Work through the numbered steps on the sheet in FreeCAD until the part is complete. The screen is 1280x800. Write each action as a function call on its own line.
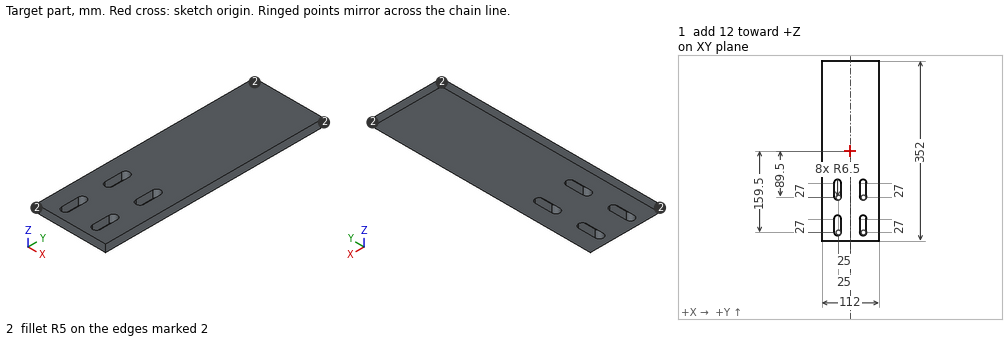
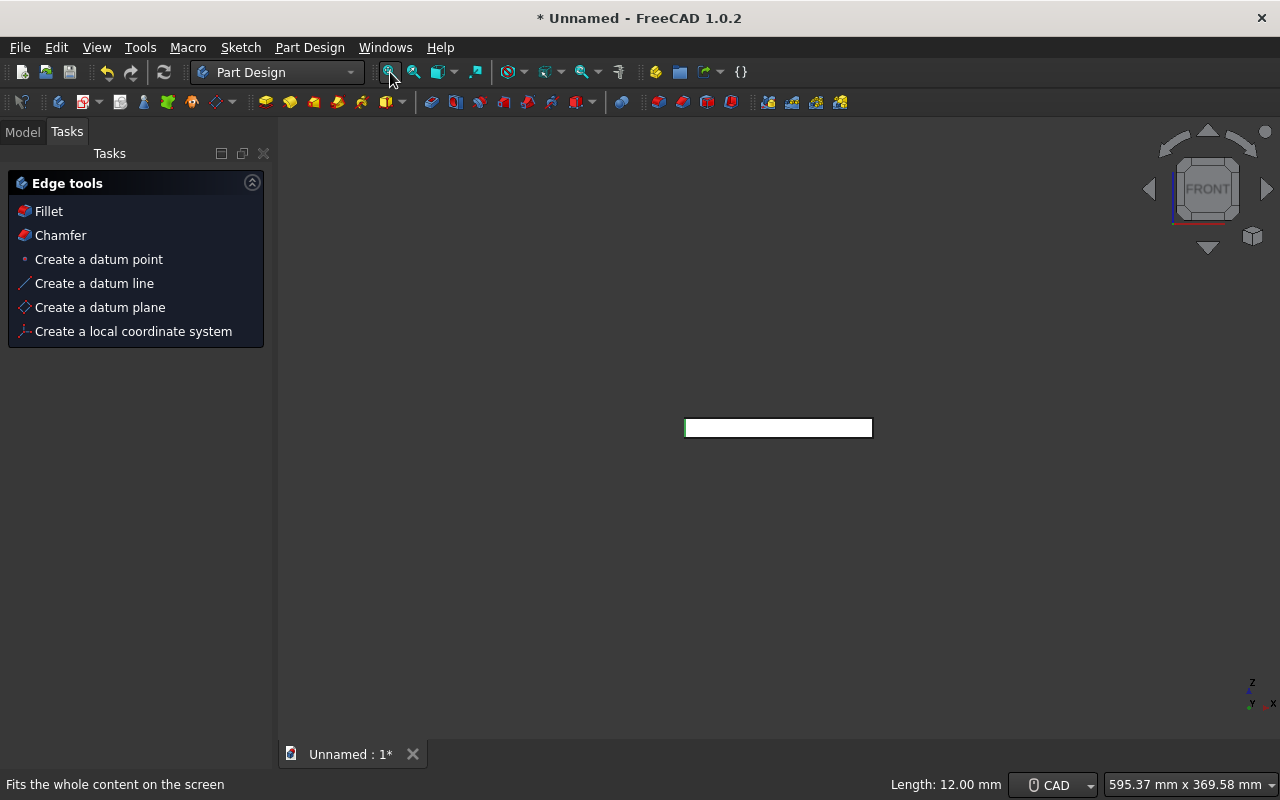
key(3)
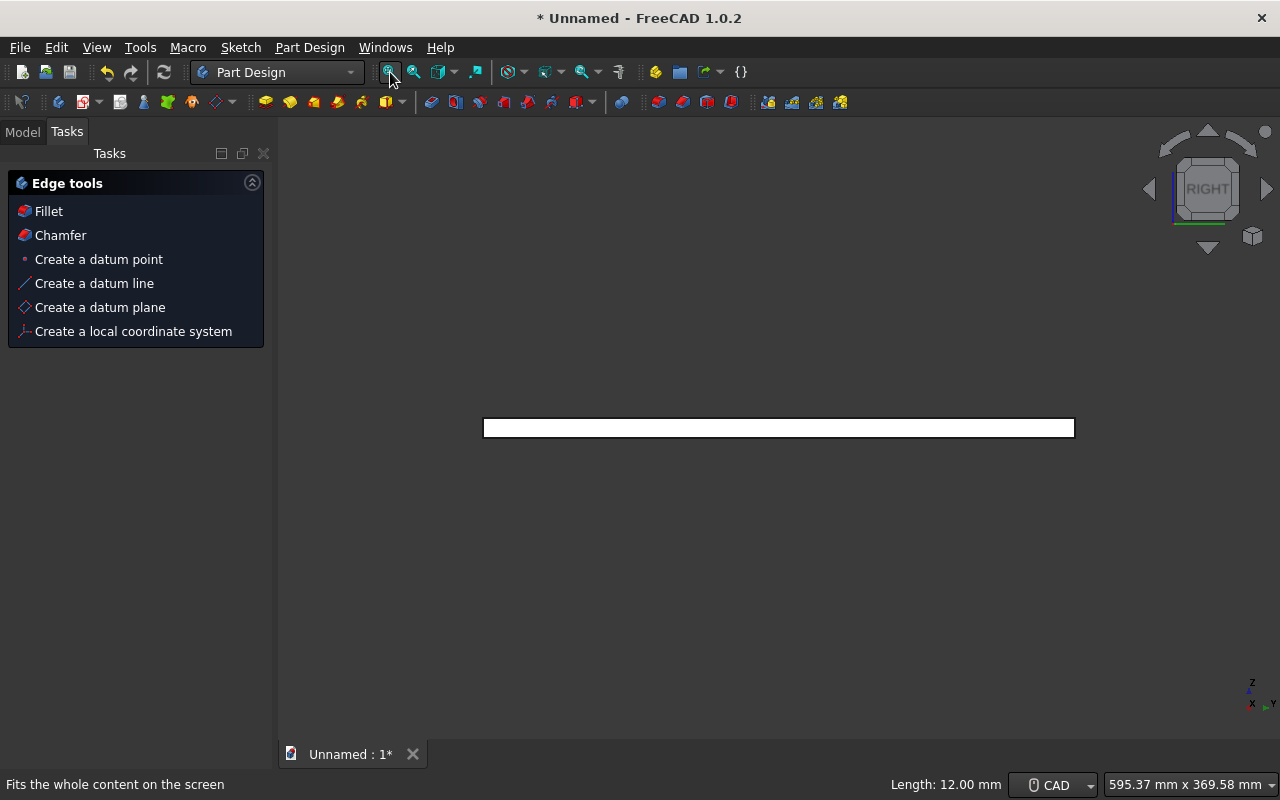
click(1075, 427, ctrl)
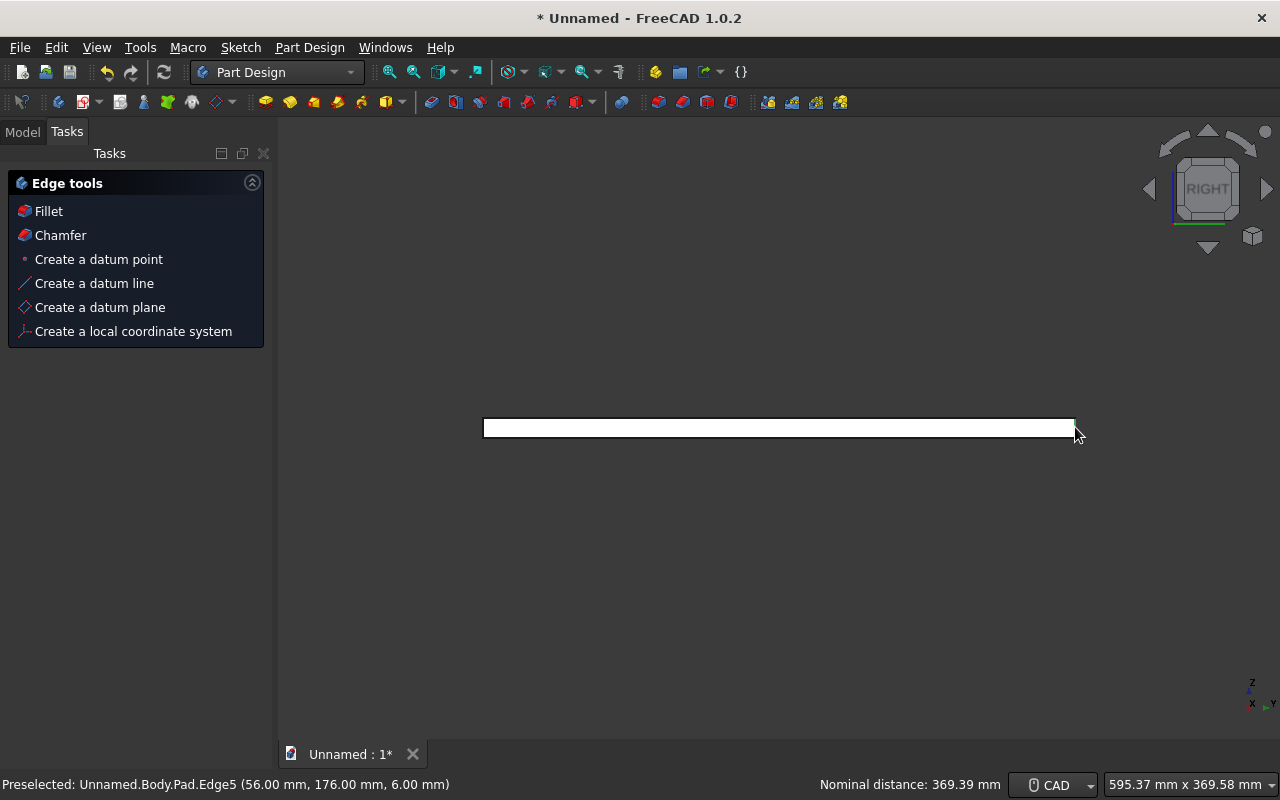
scroll(1075, 427, up, 4)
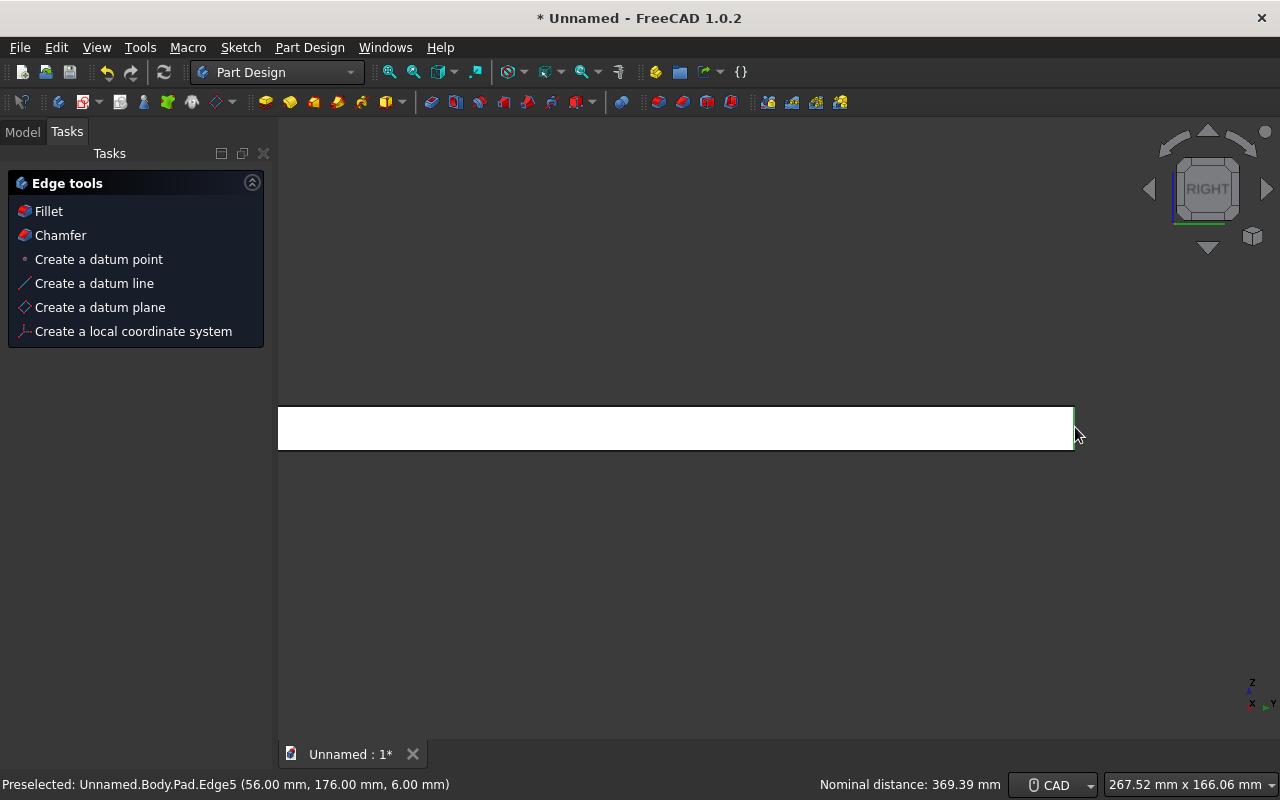
click(390, 72)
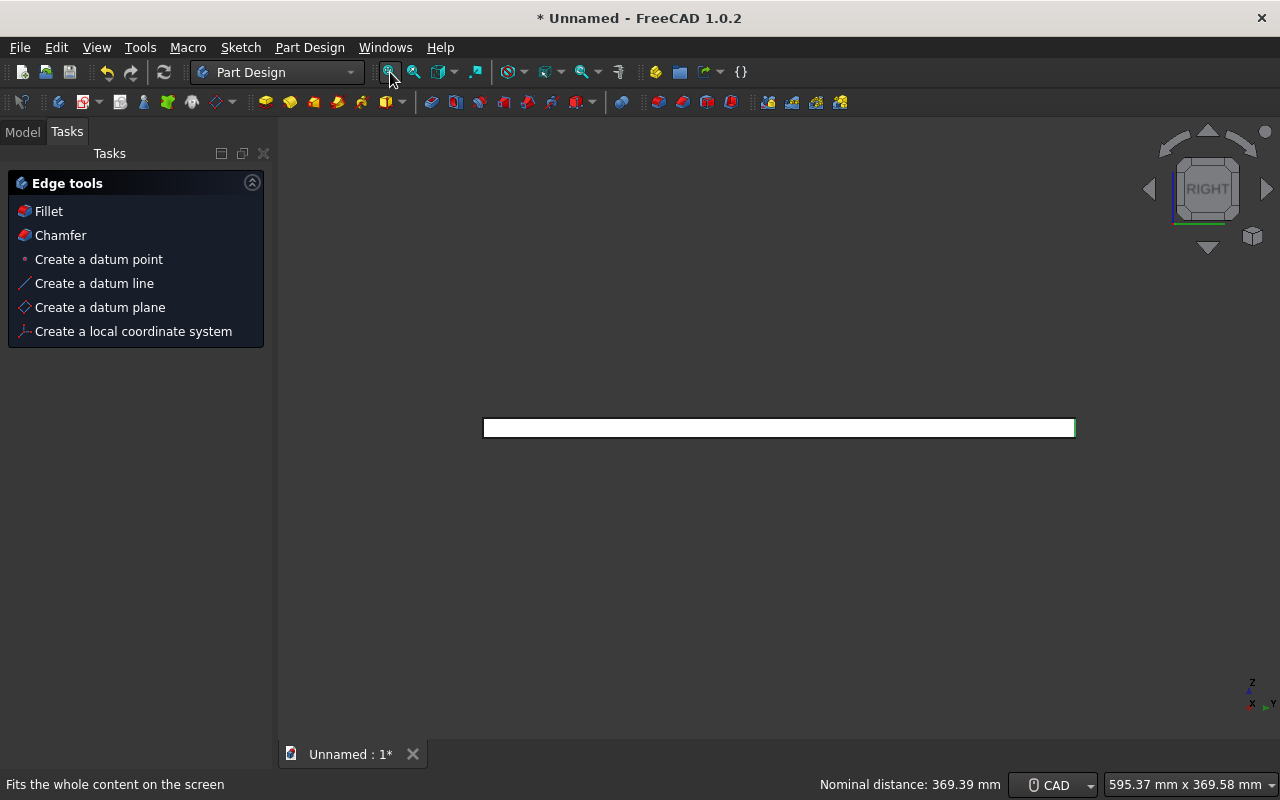
key(5)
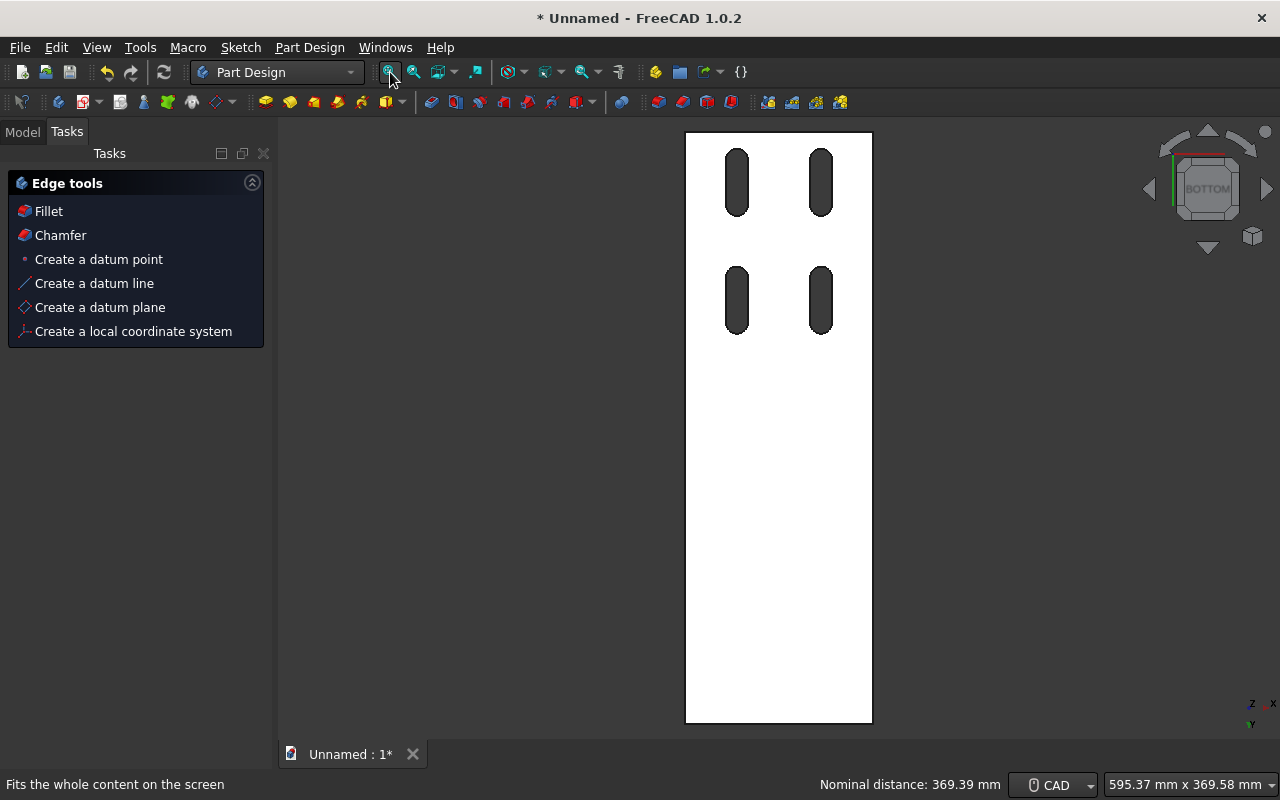
key(4)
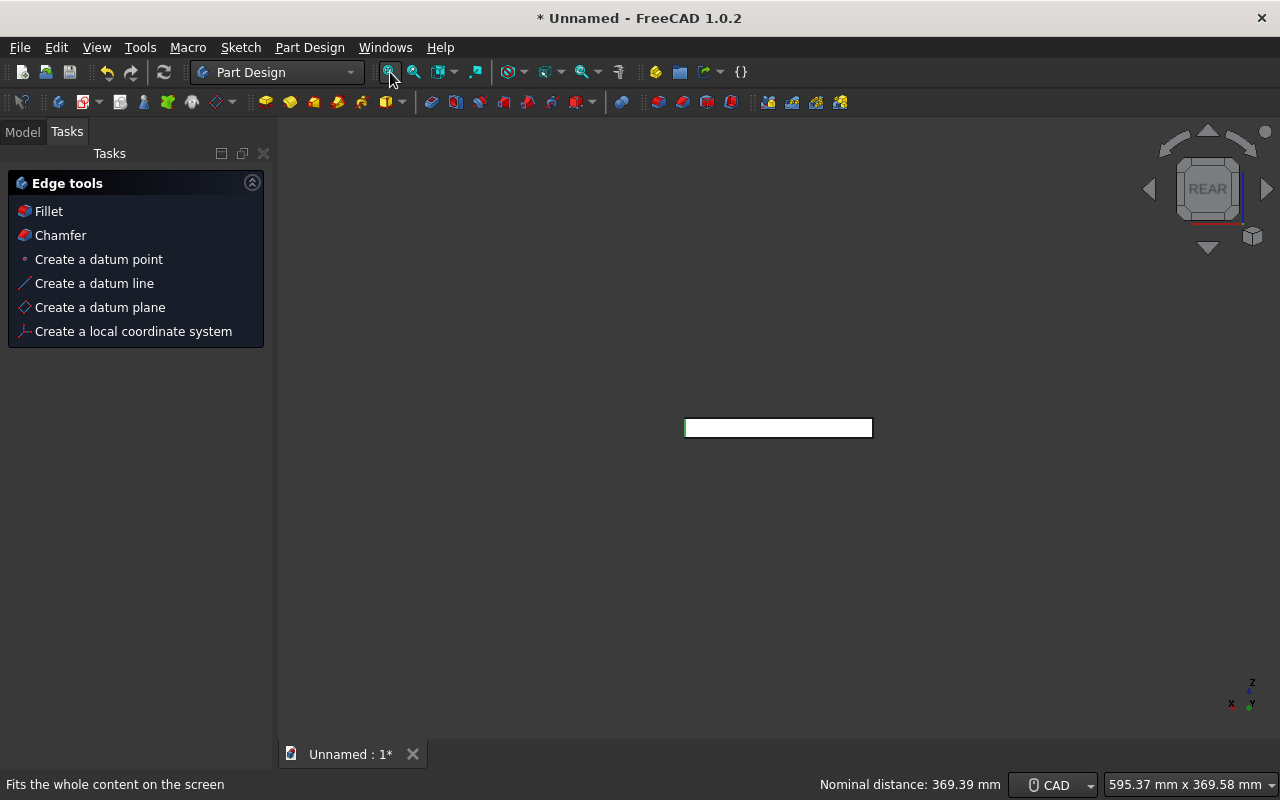
click(390, 72)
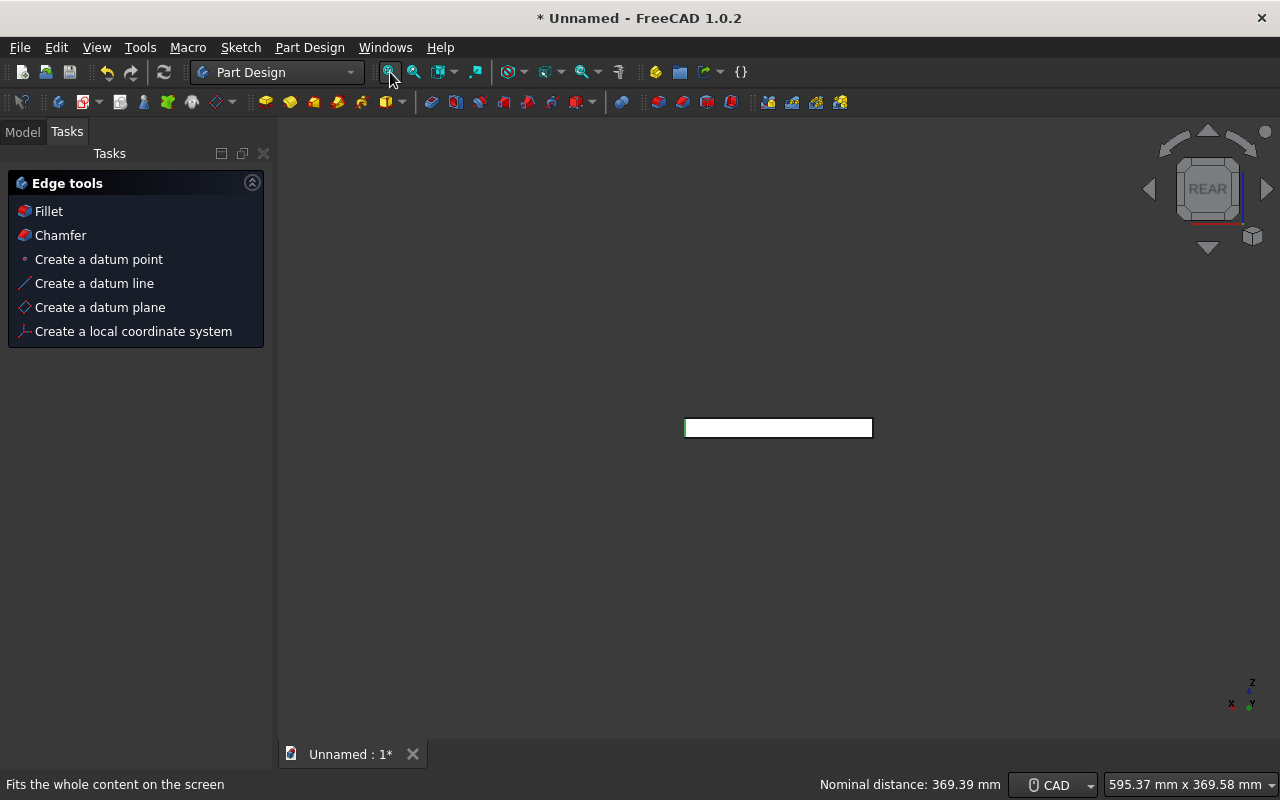
click(873, 427, ctrl)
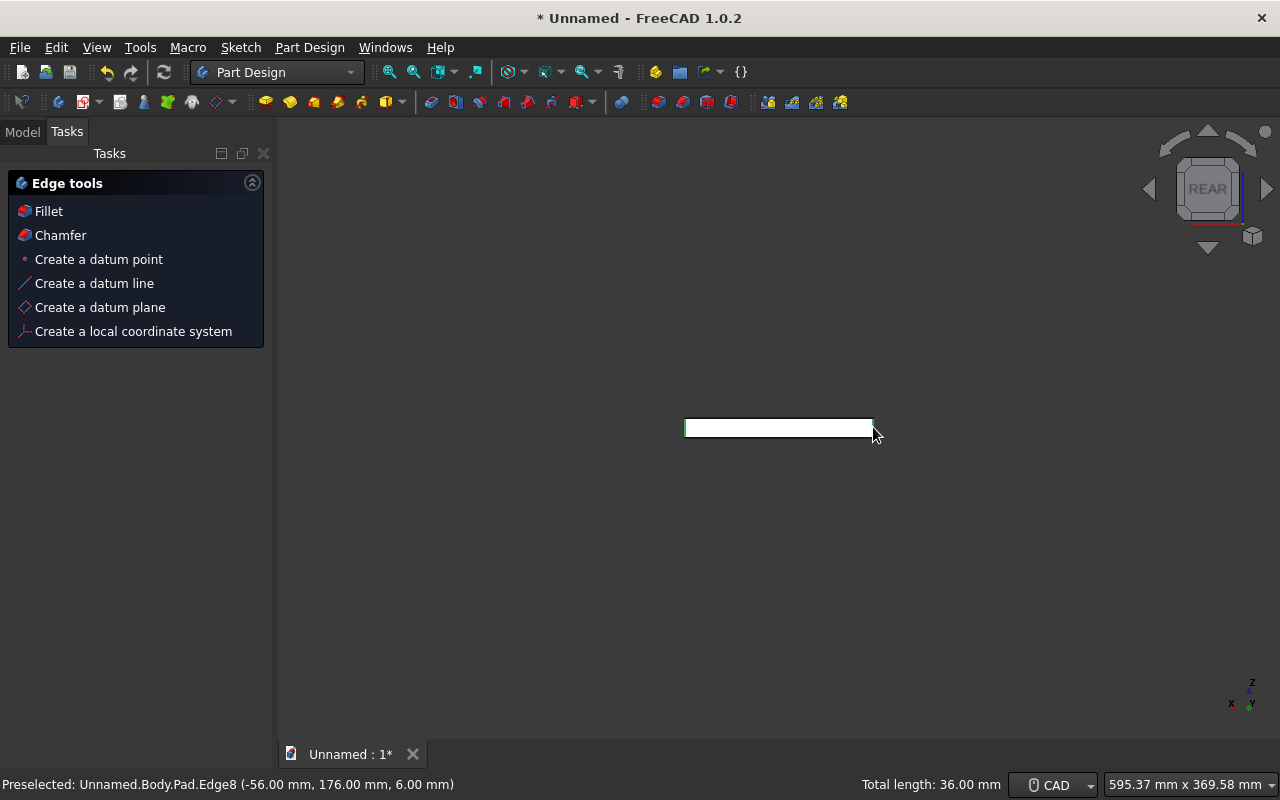
click(660, 102)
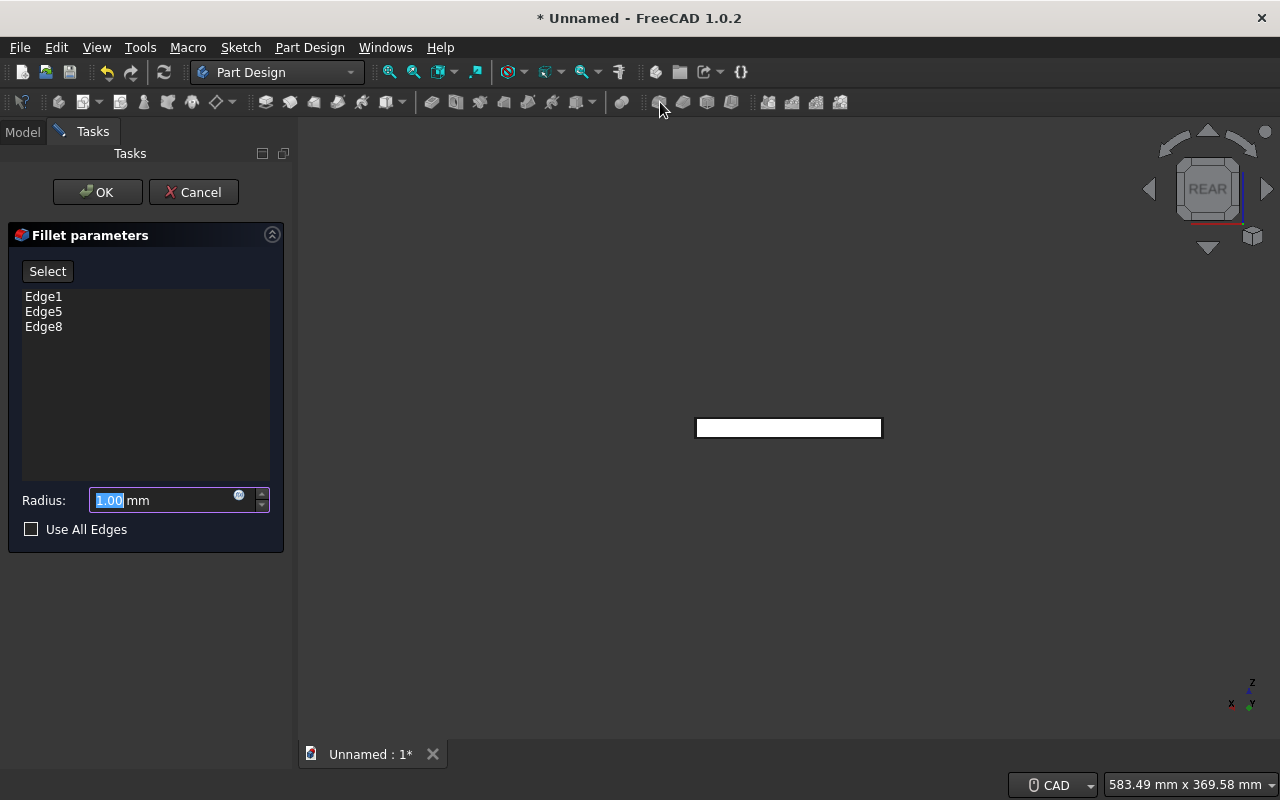
text(5)
key(Tab)